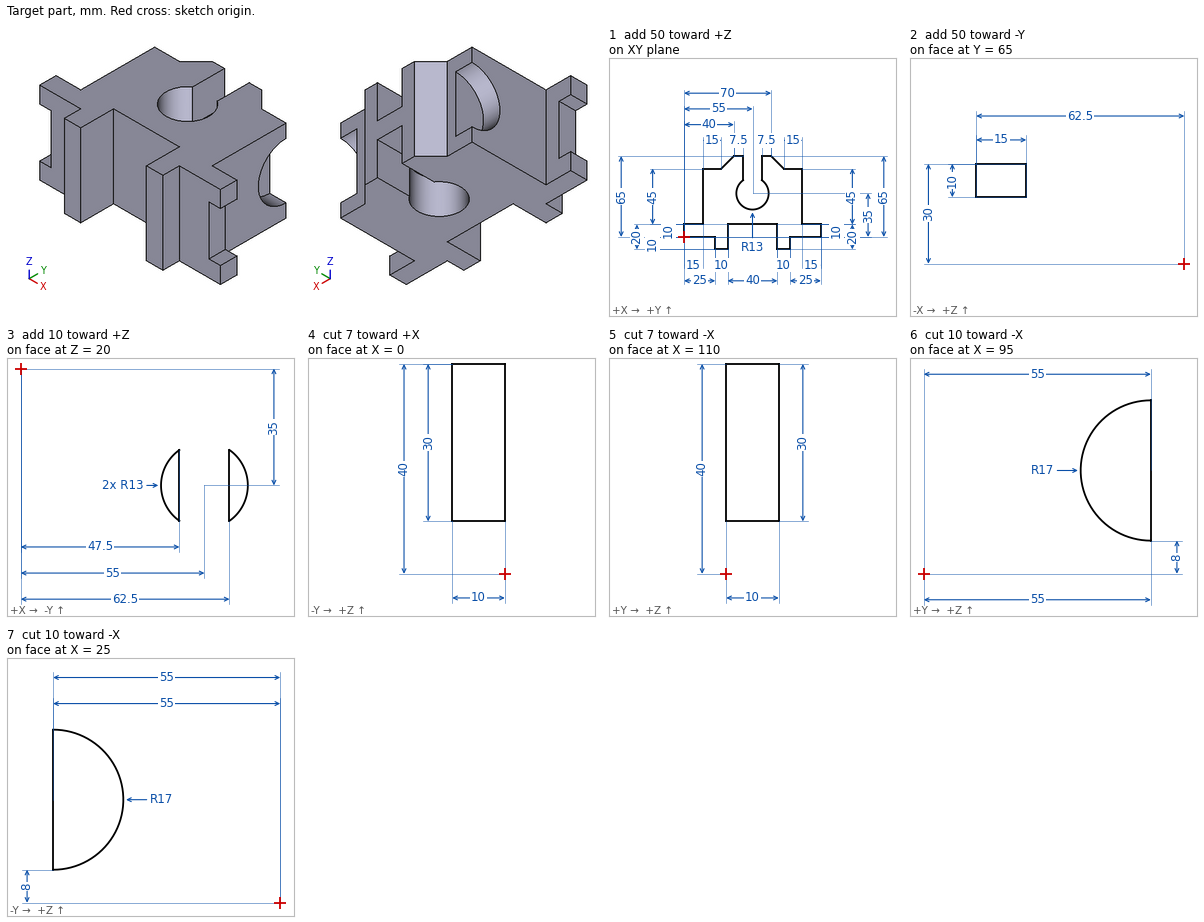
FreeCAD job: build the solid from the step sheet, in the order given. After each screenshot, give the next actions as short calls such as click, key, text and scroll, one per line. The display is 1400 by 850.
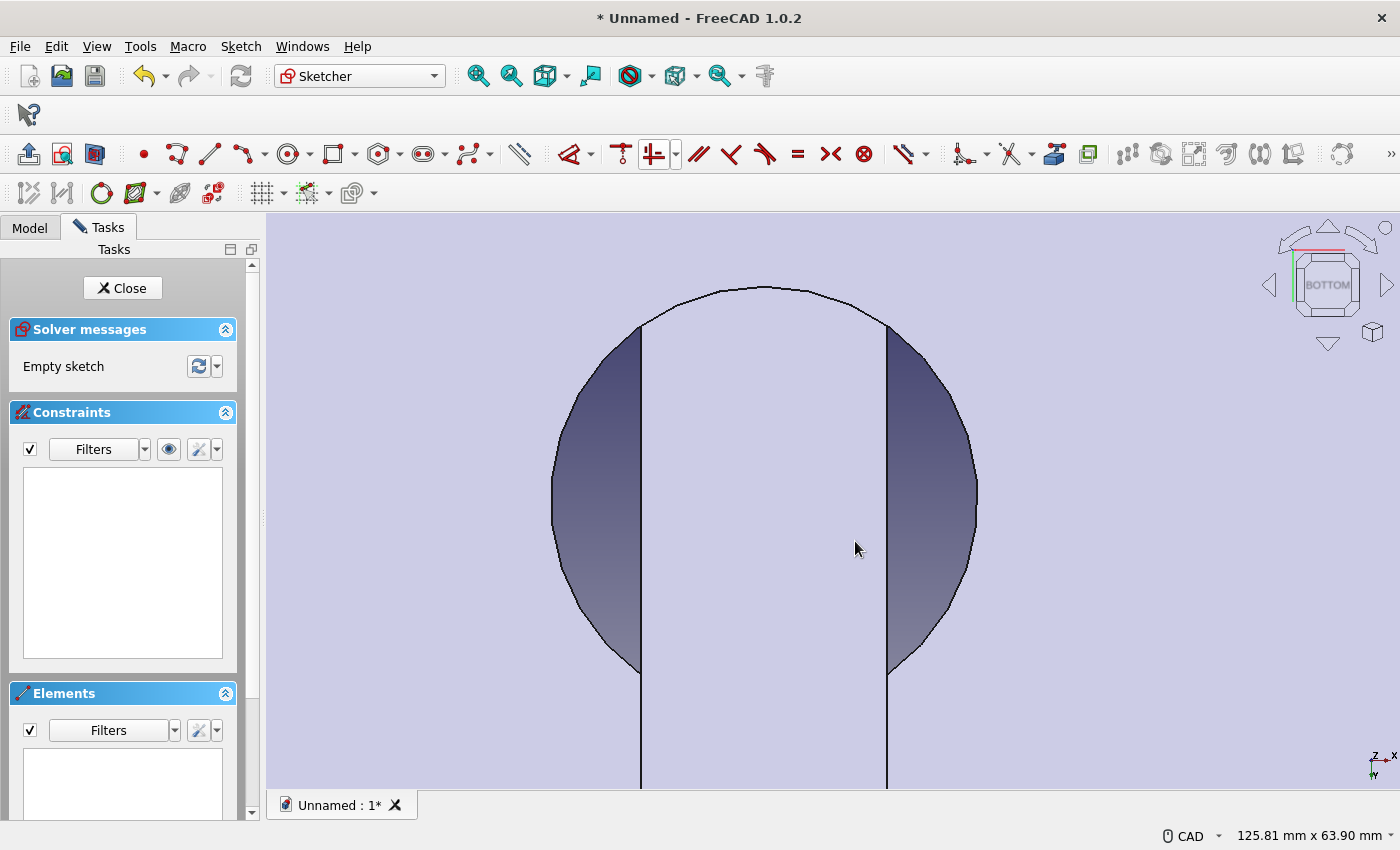
click(210, 154)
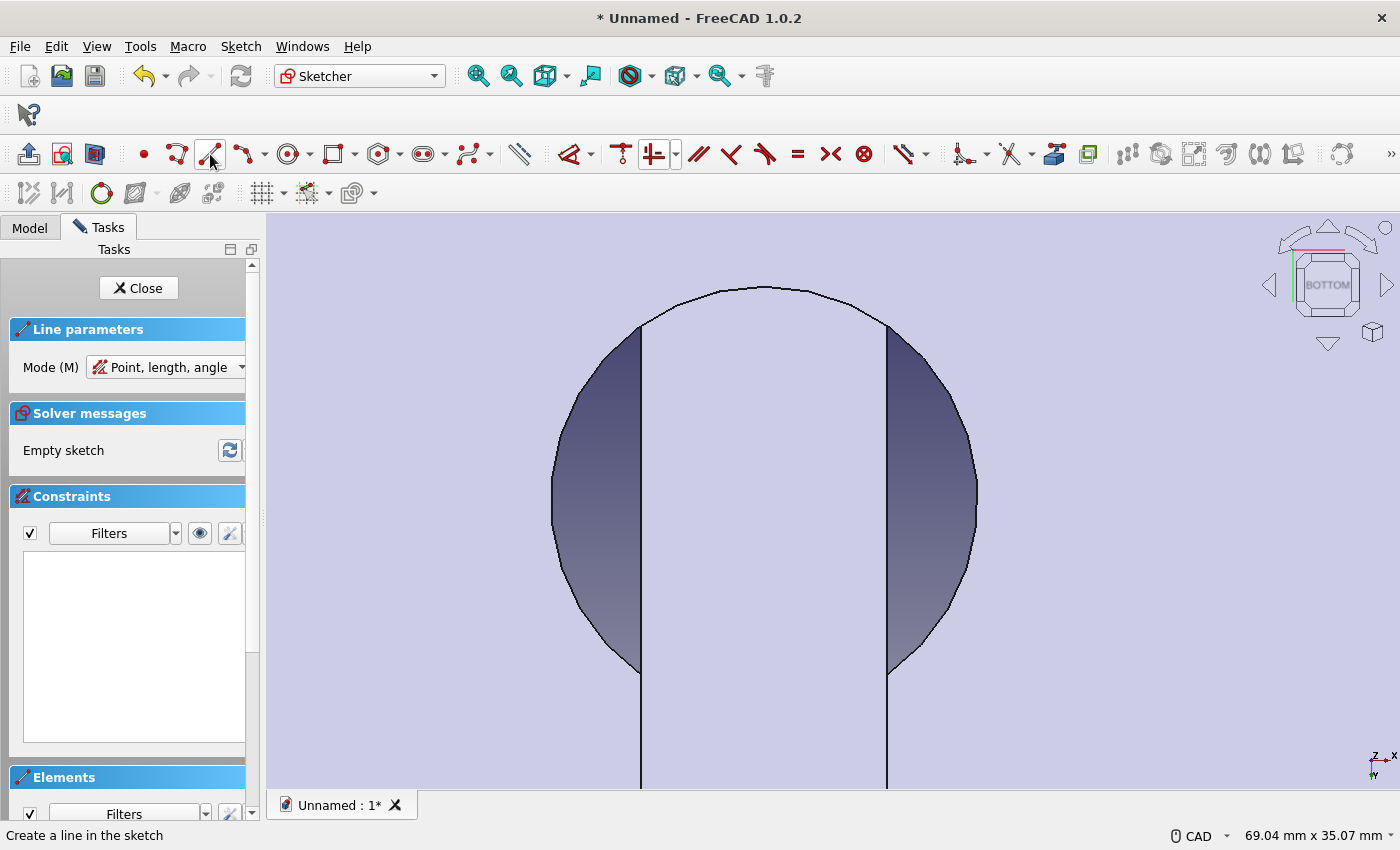
click(641, 326)
click(641, 675)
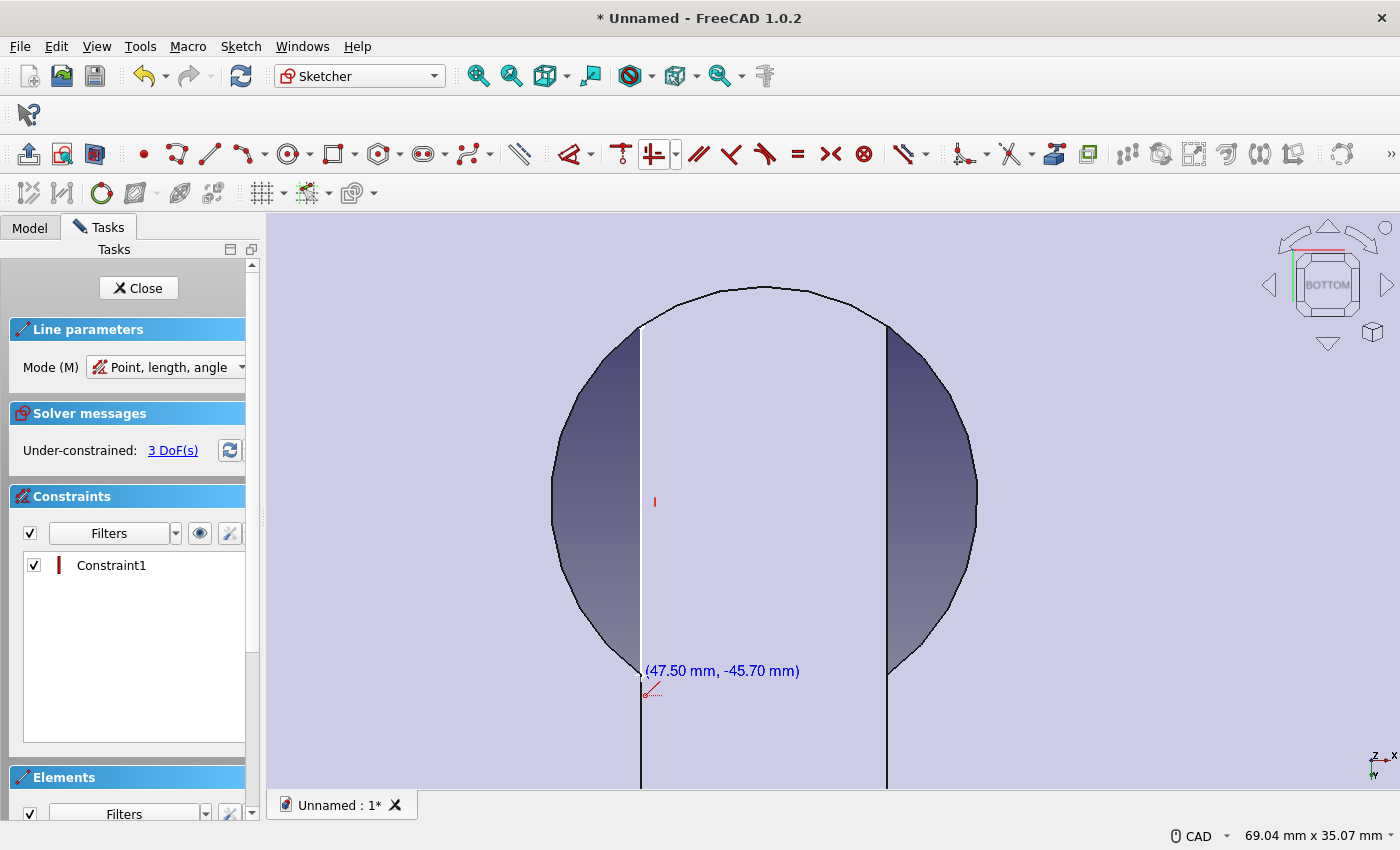
click(242, 154)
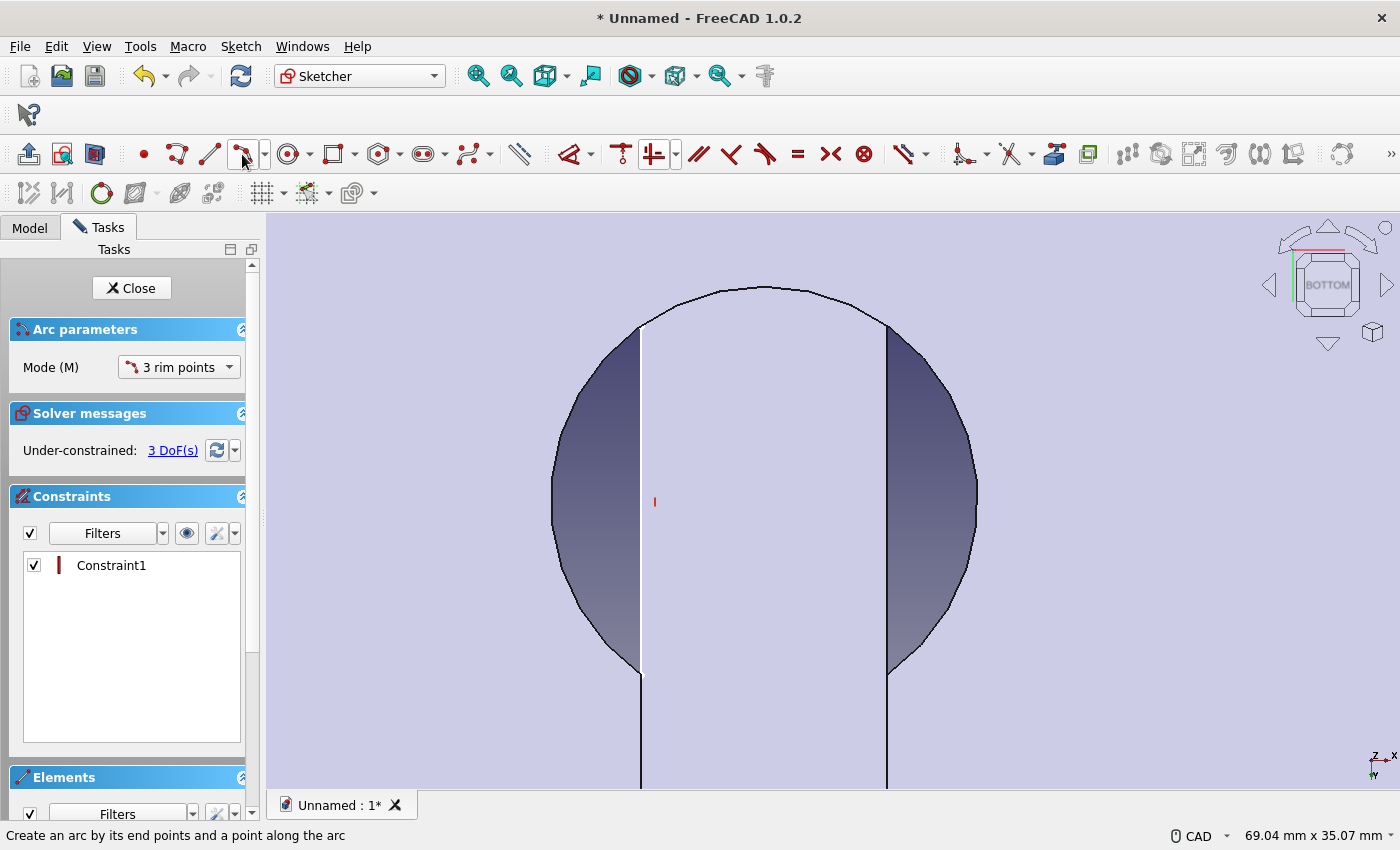
click(641, 676)
click(641, 327)
click(551, 500)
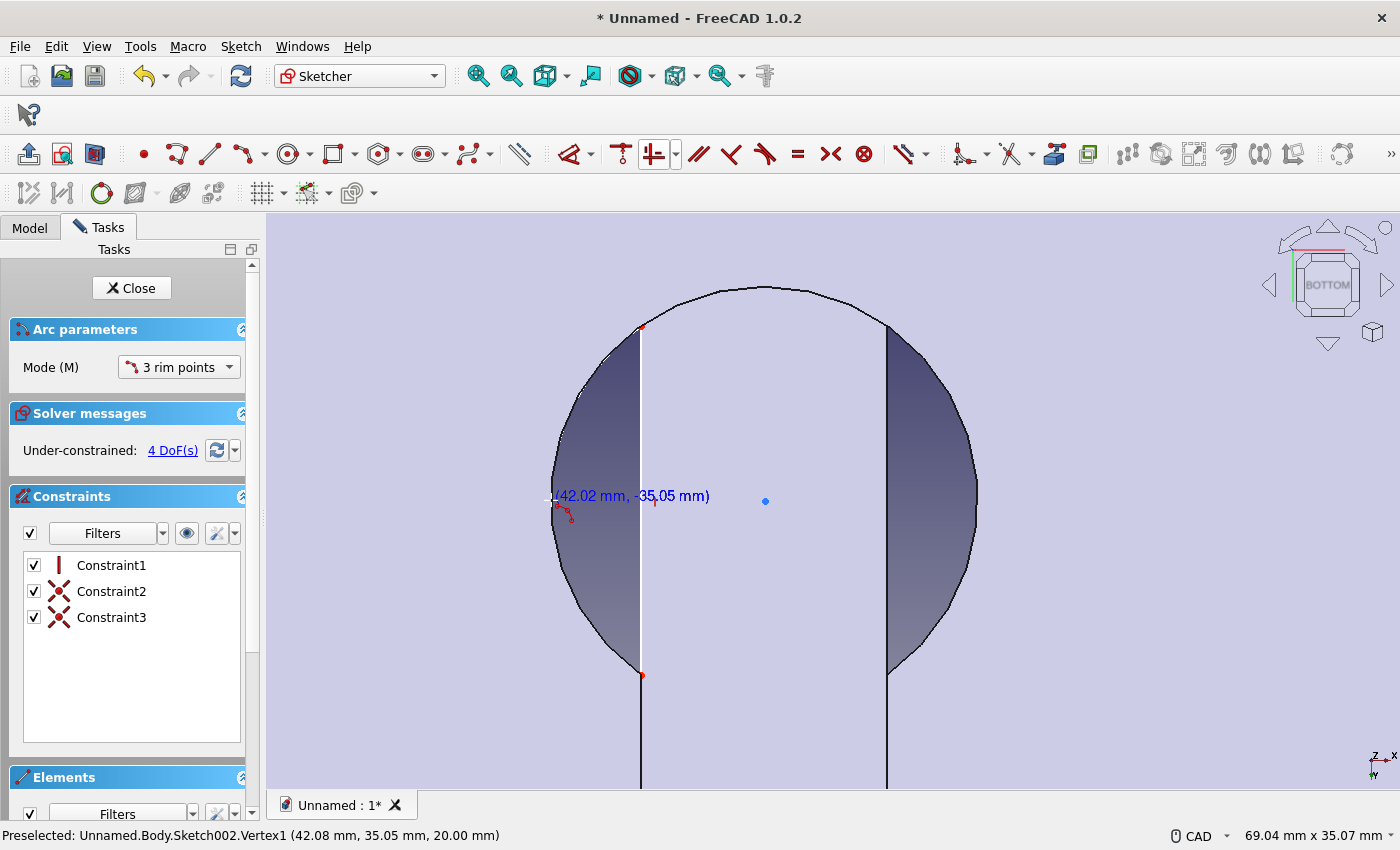
click(210, 154)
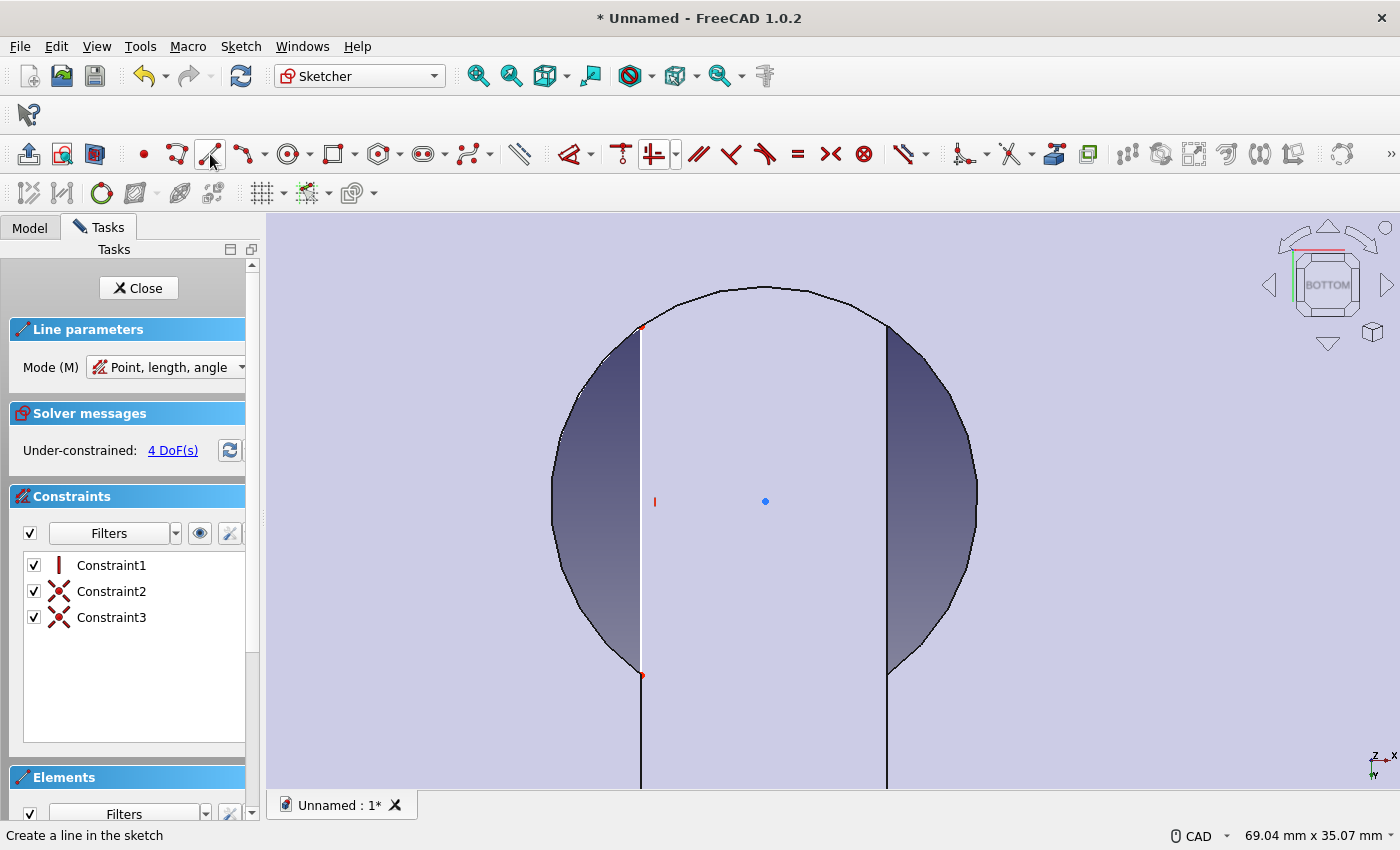
click(887, 675)
click(887, 326)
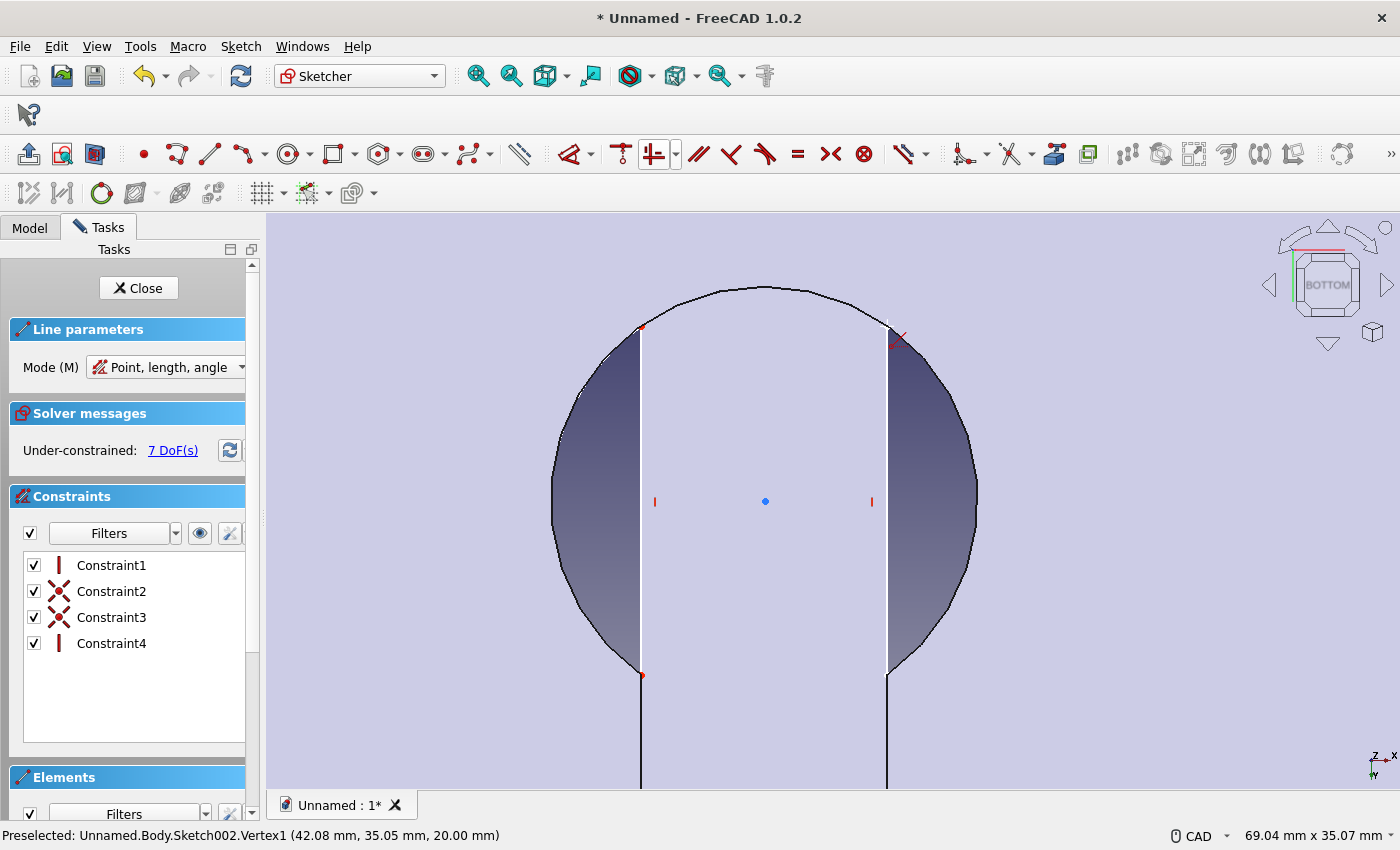
click(242, 154)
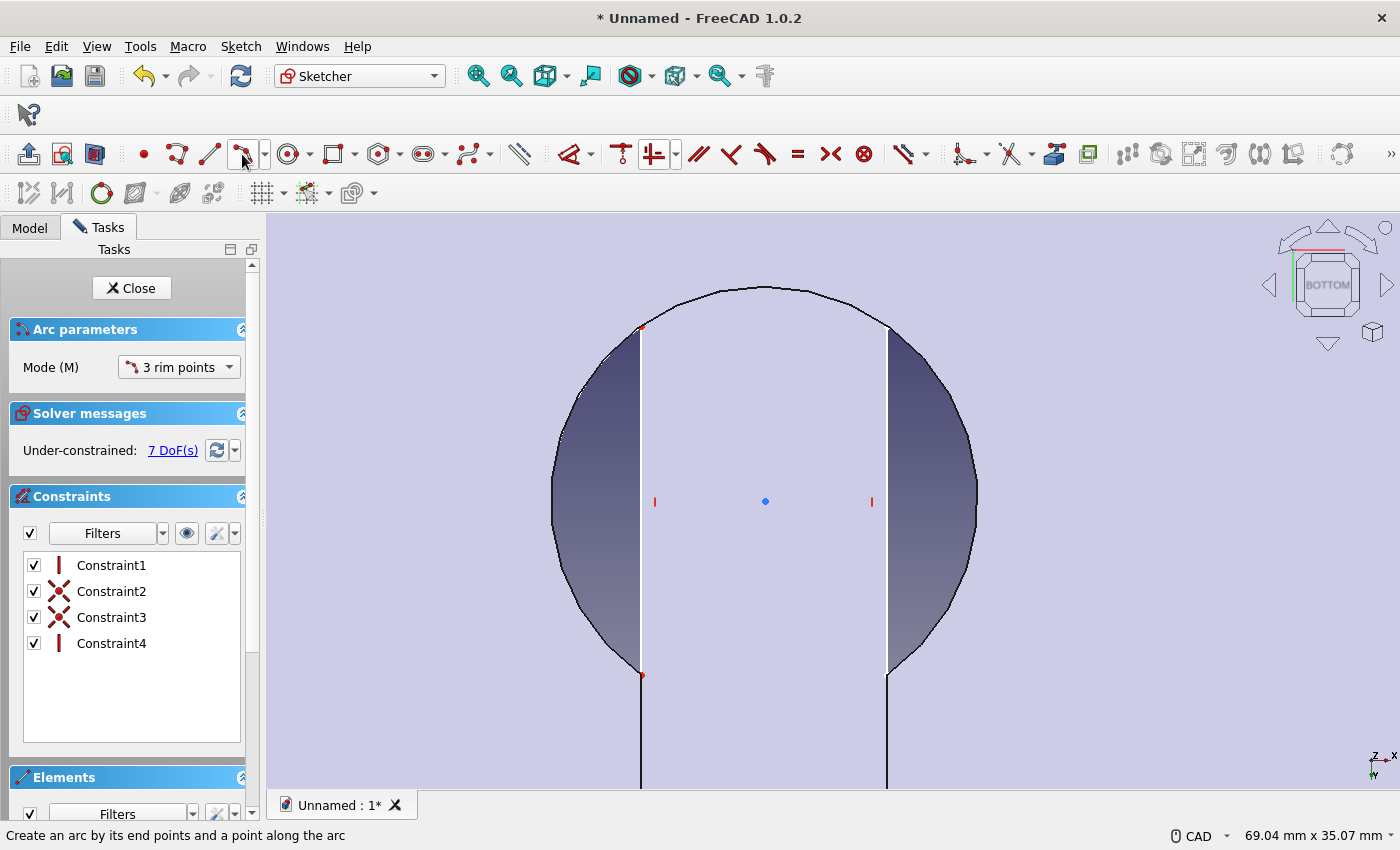
click(887, 327)
click(887, 676)
click(978, 500)
key(Escape)